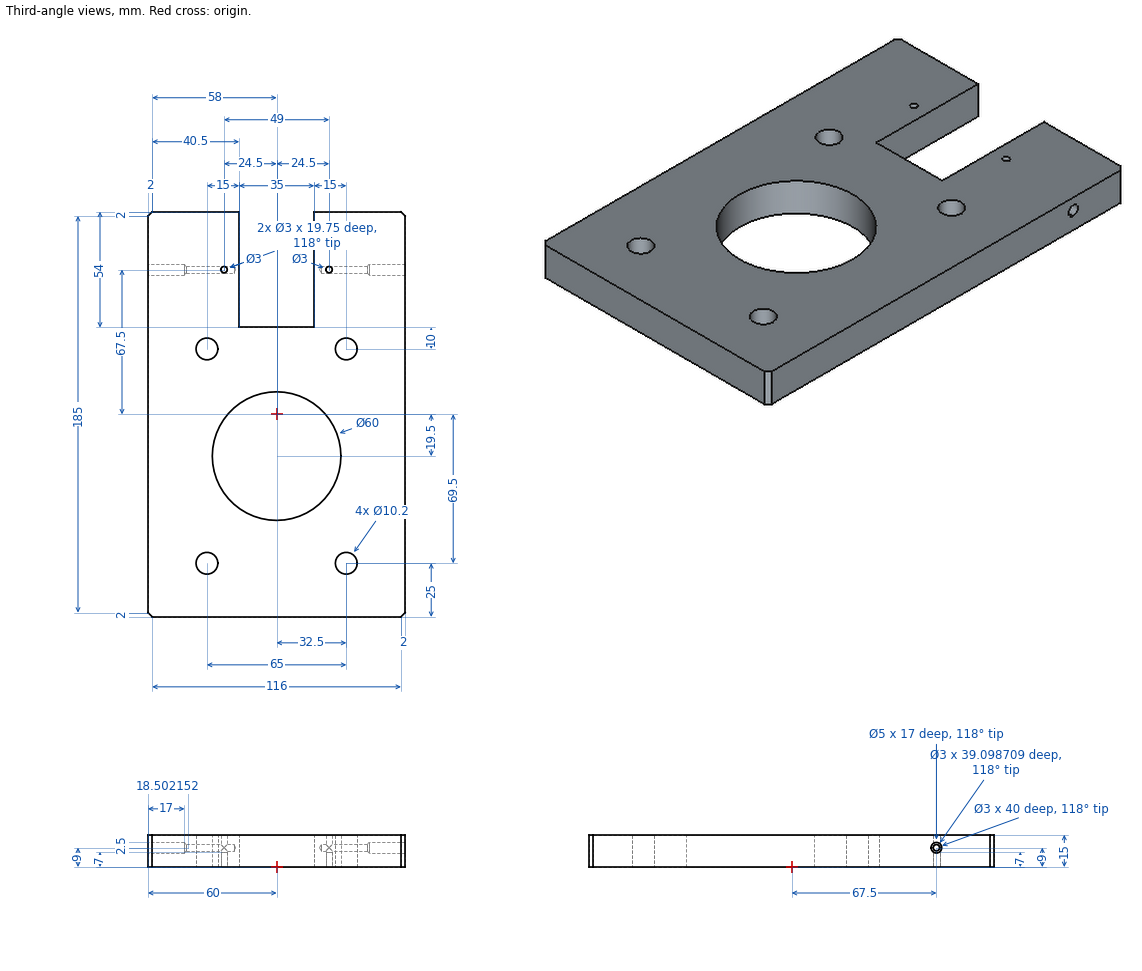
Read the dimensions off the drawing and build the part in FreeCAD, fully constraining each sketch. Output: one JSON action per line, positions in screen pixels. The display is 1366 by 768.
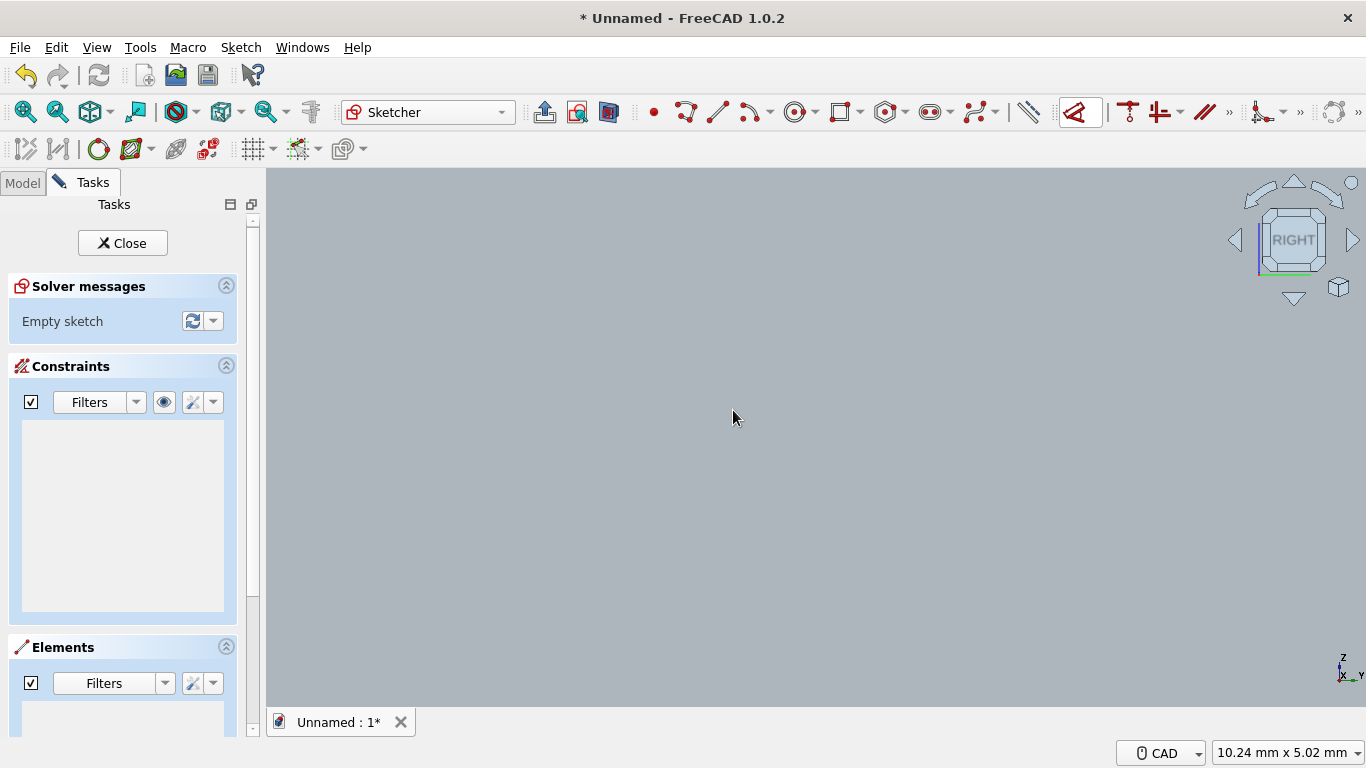
{"action": "key", "text": "g c"}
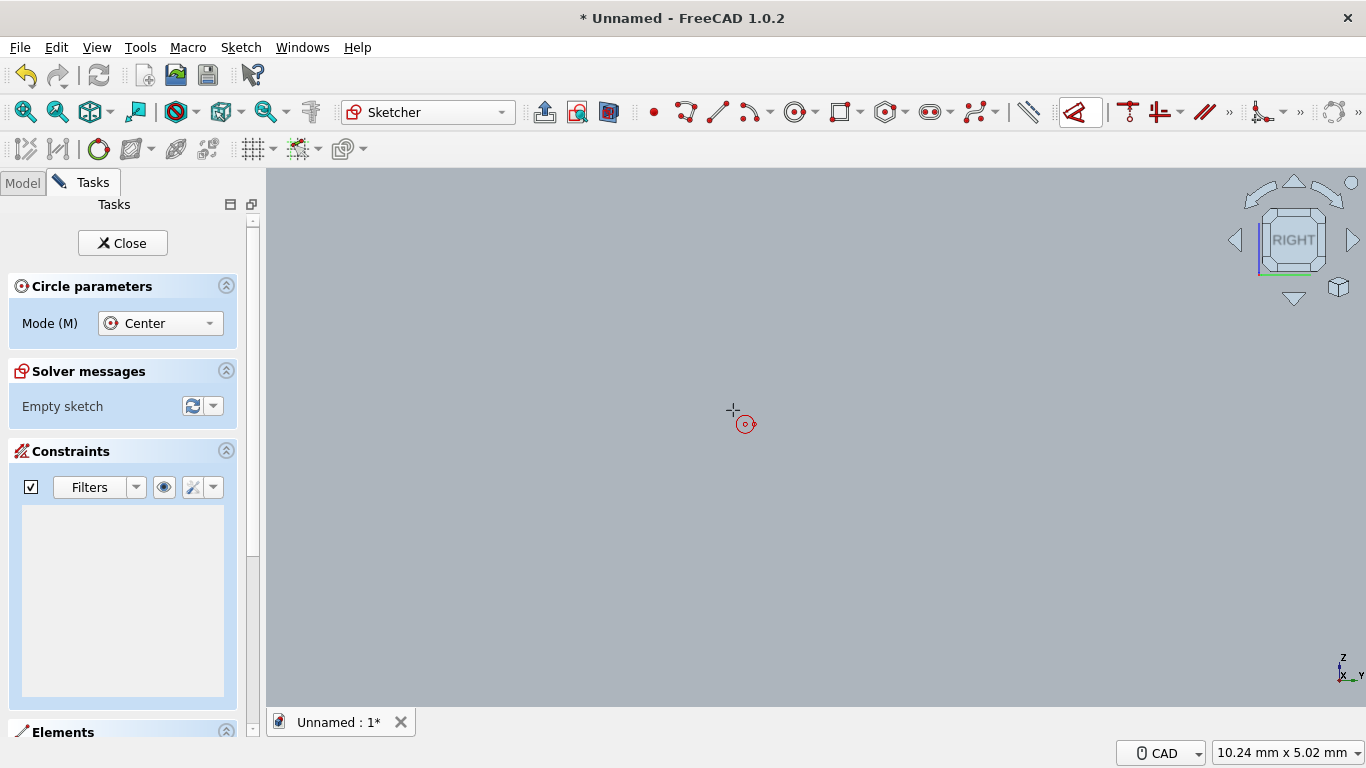
{"action": "left_click", "coordinate": [747, 437]}
{"action": "mouse_move", "coordinate": [861, 323]}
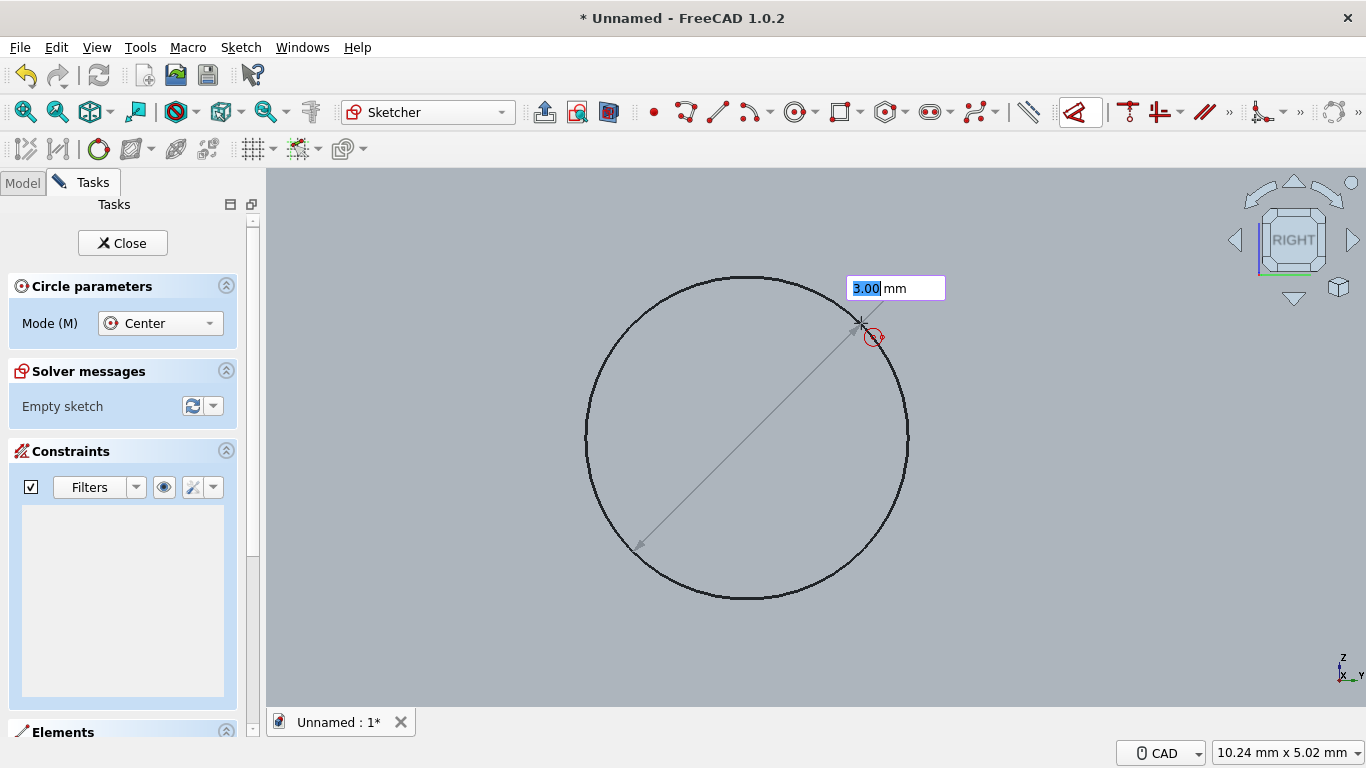
{"action": "type", "text": "3"}
{"action": "key", "text": "Return"}
{"action": "key", "text": "Escape"}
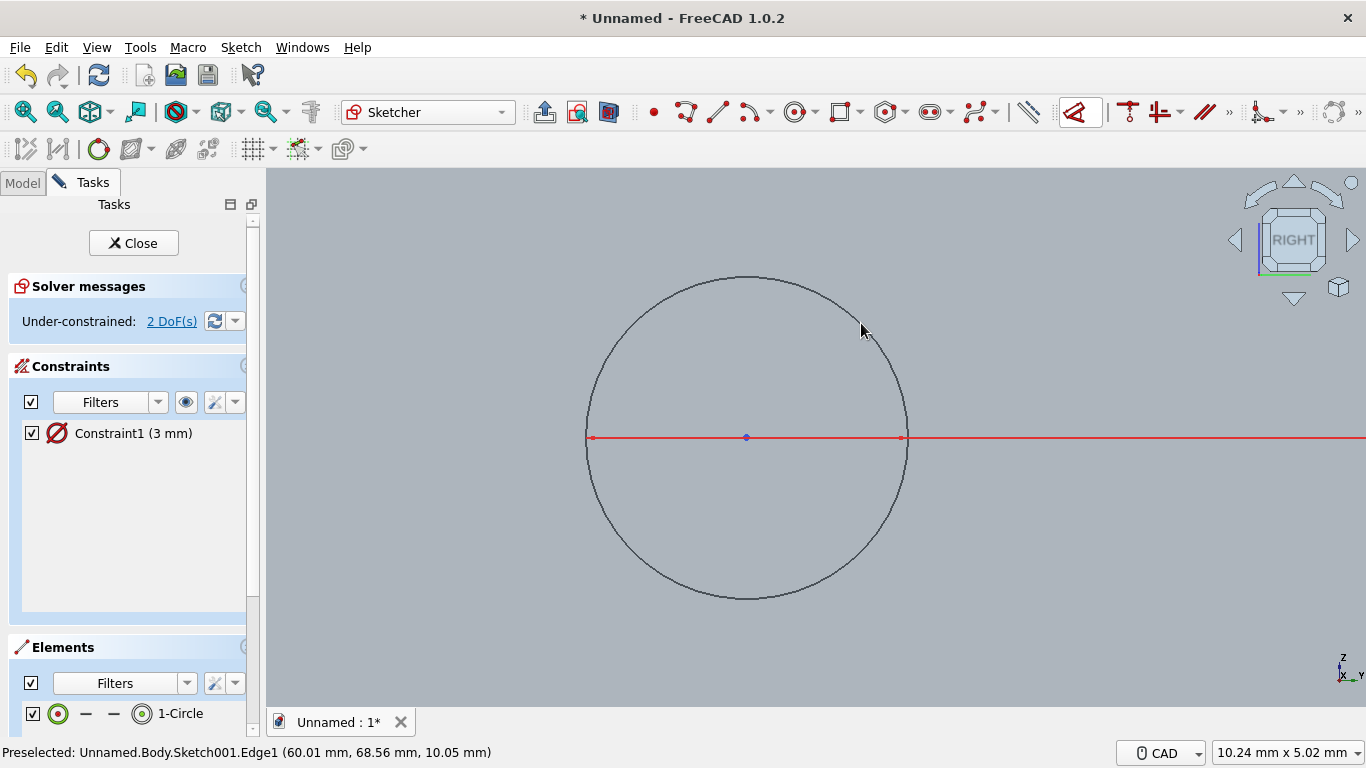
{"action": "left_click", "coordinate": [747, 438]}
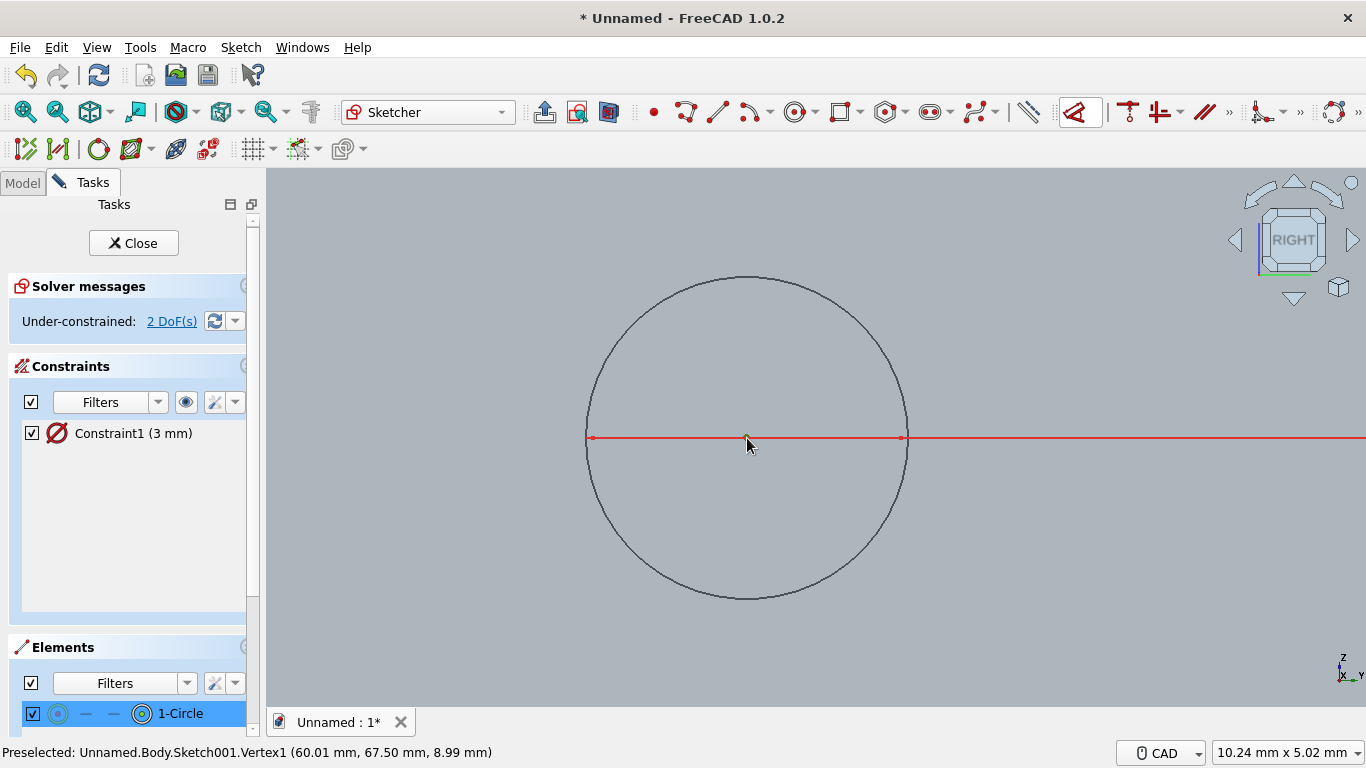
{"action": "left_click", "coordinate": [1096, 112]}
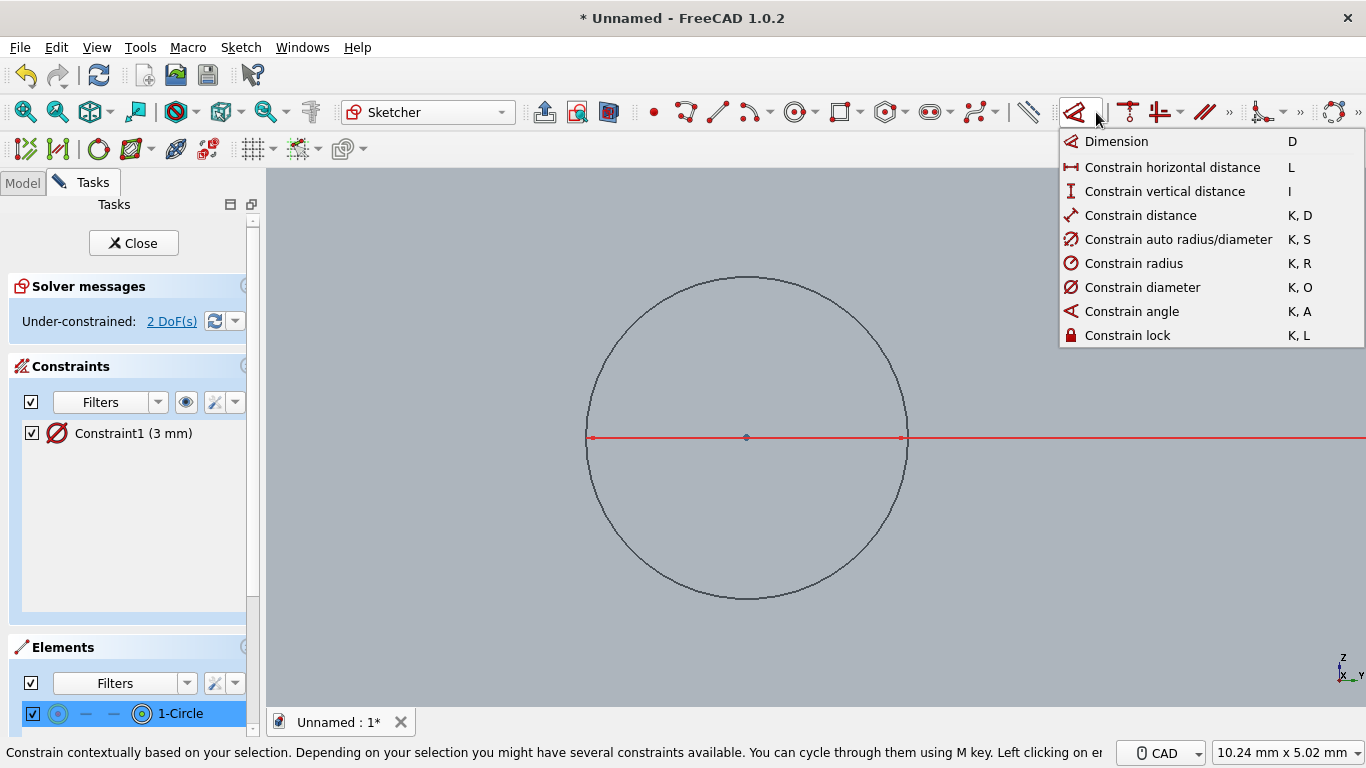
{"action": "left_click", "coordinate": [1212, 191]}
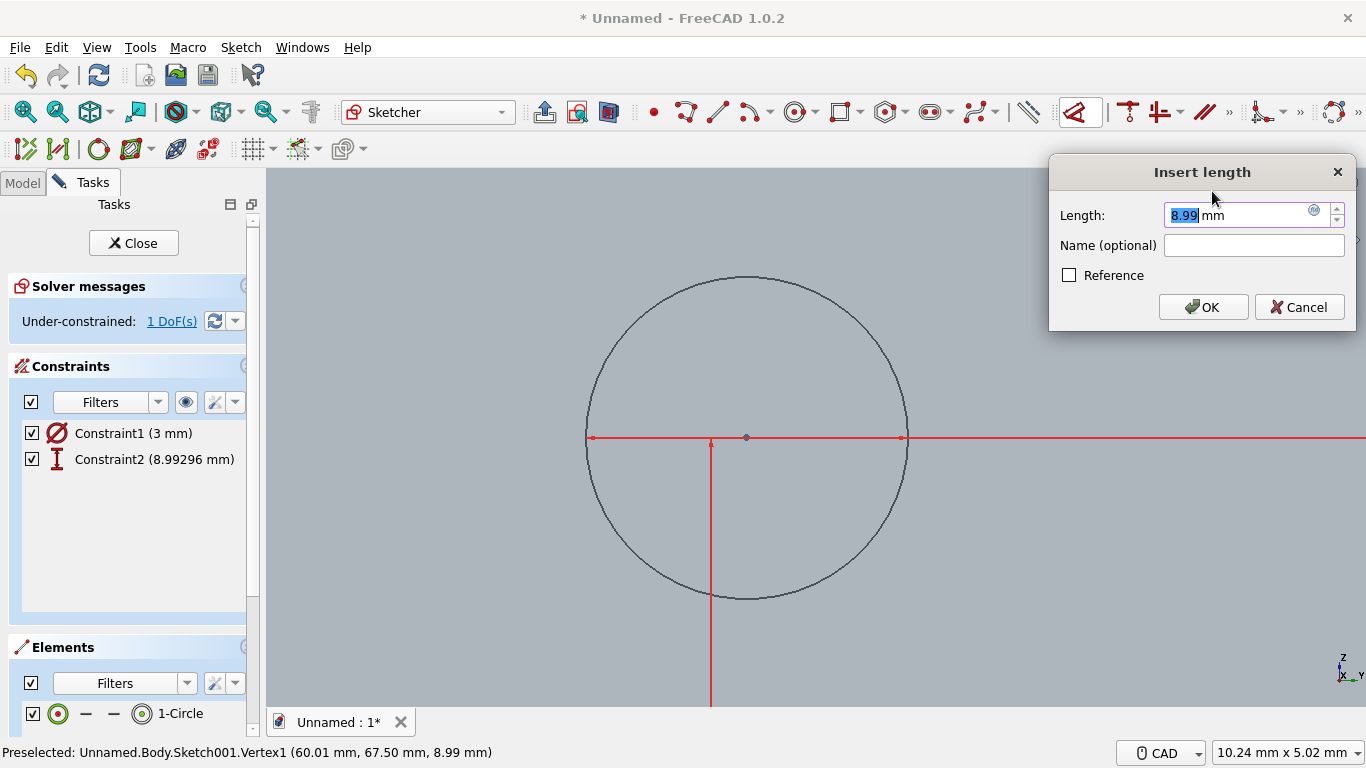
{"action": "type", "text": "9"}
{"action": "key", "text": "Return"}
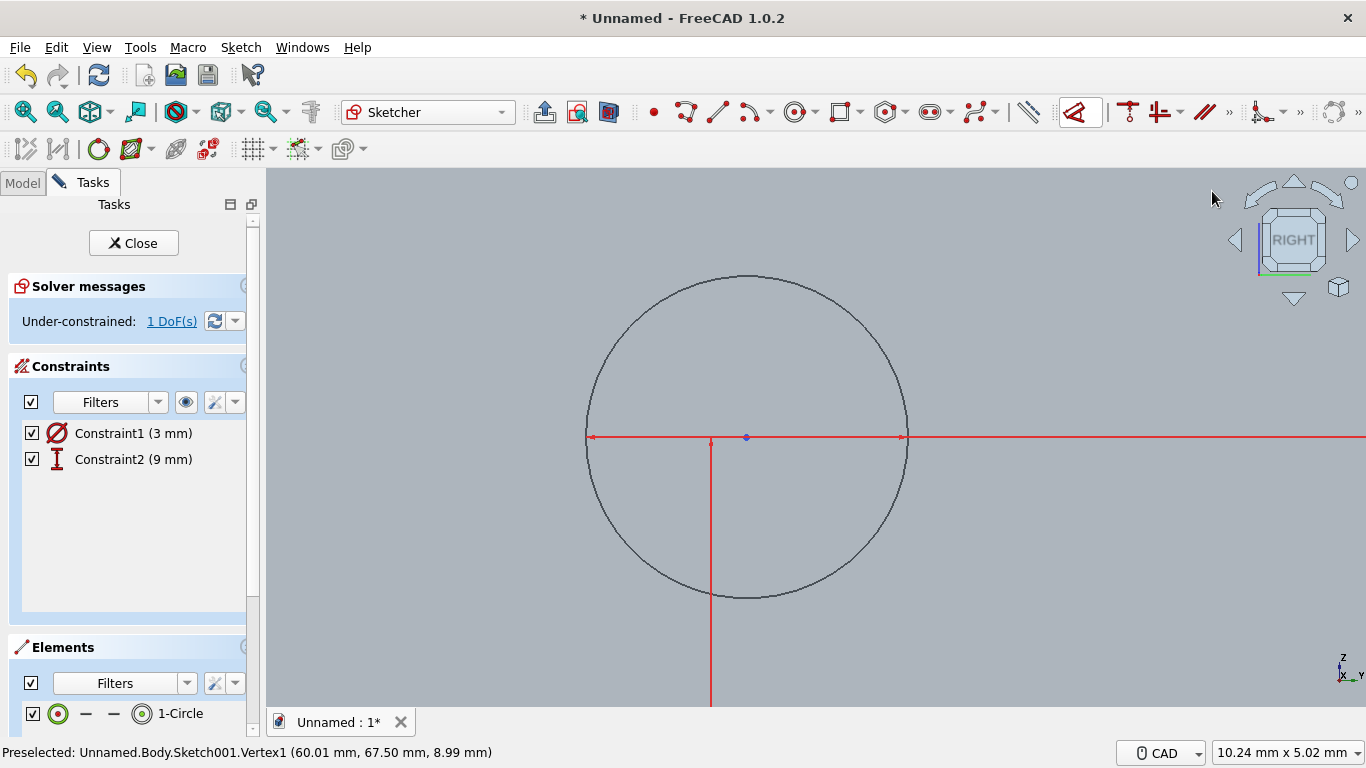
{"action": "left_click", "coordinate": [747, 437]}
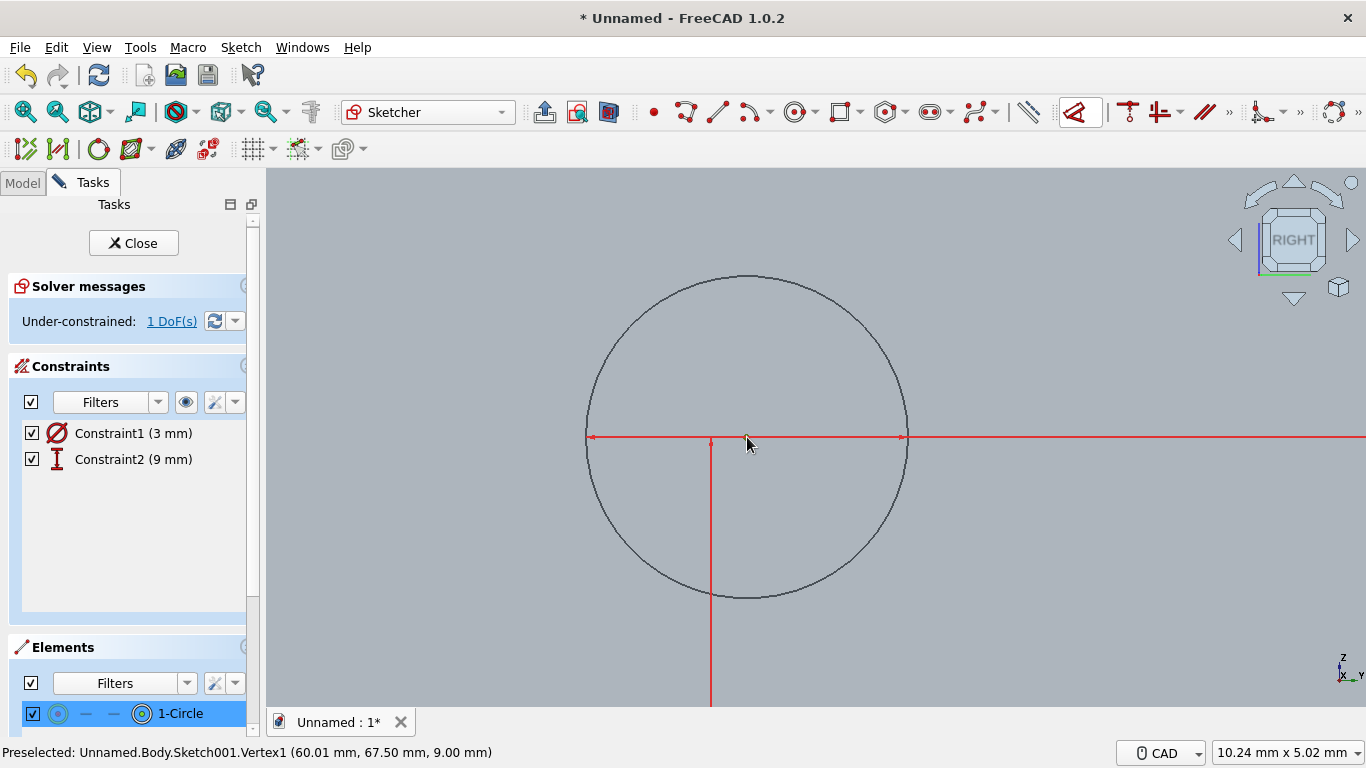
{"action": "left_click", "coordinate": [1096, 112]}